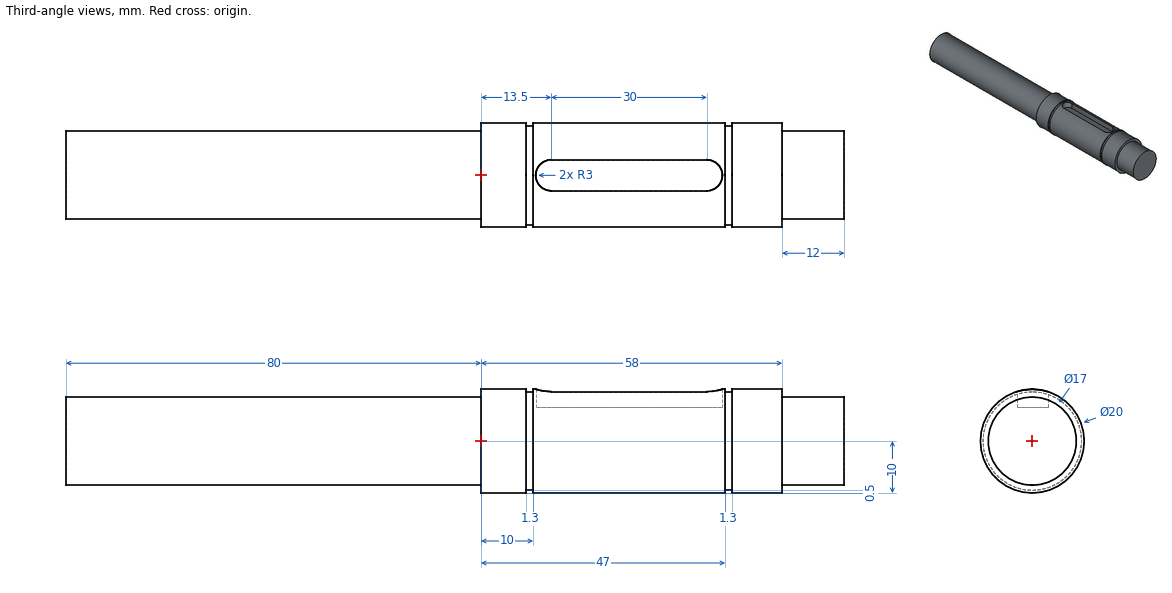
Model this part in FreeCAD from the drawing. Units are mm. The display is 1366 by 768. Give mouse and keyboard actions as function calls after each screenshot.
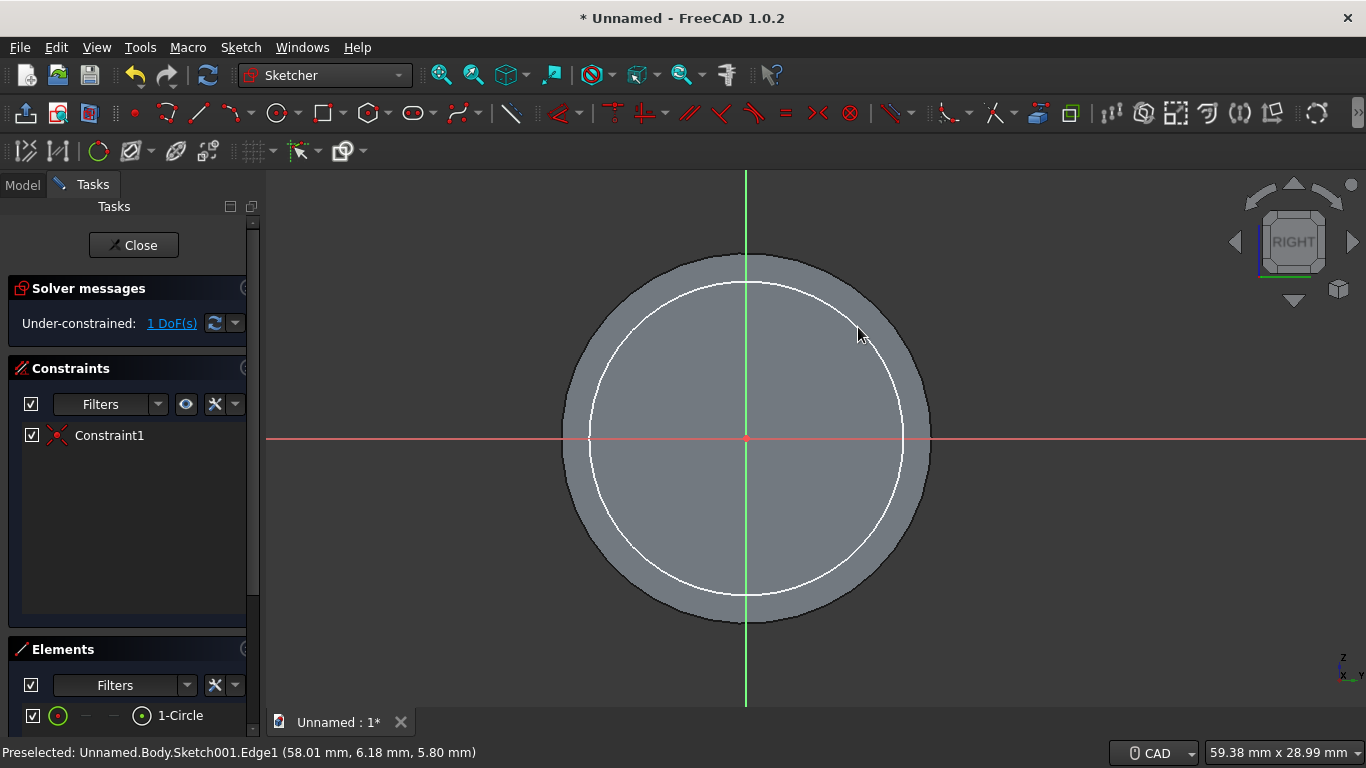
click(558, 114)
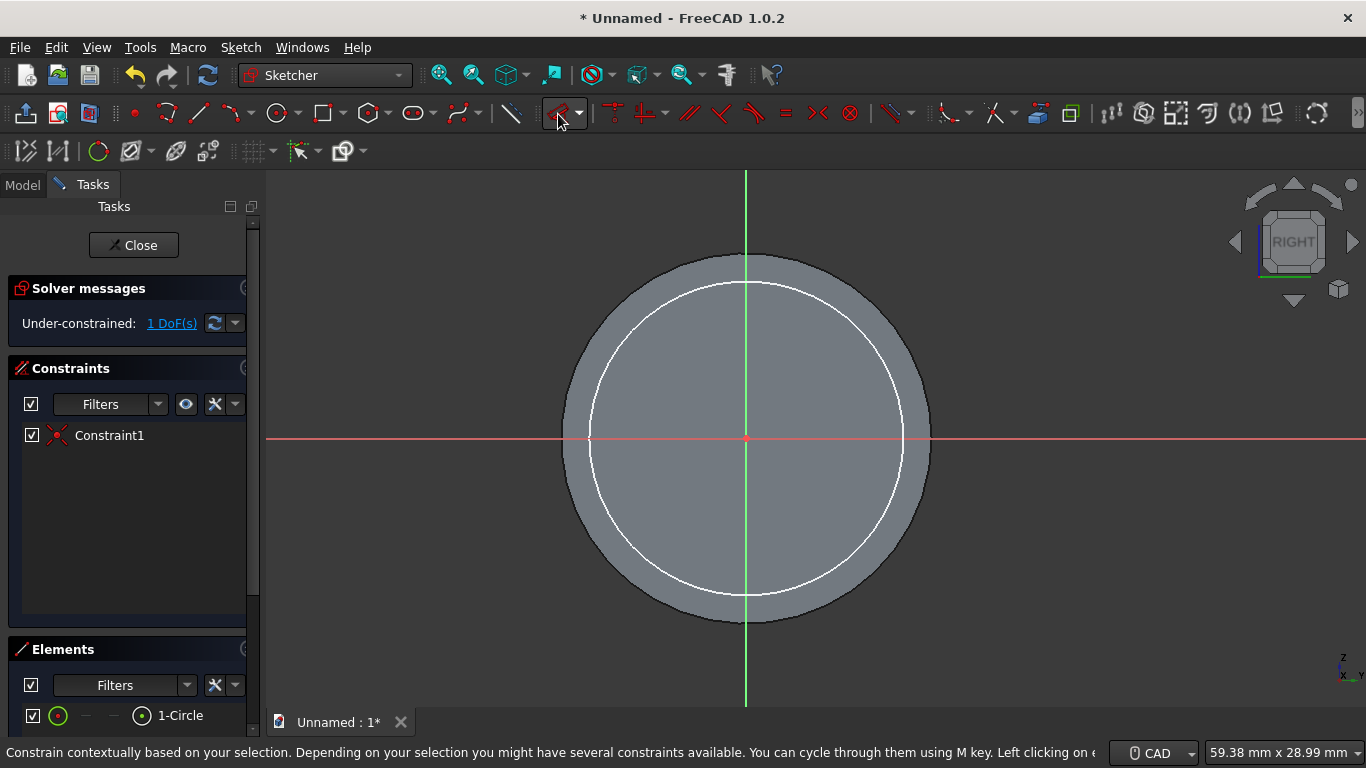
click(857, 327)
click(880, 304)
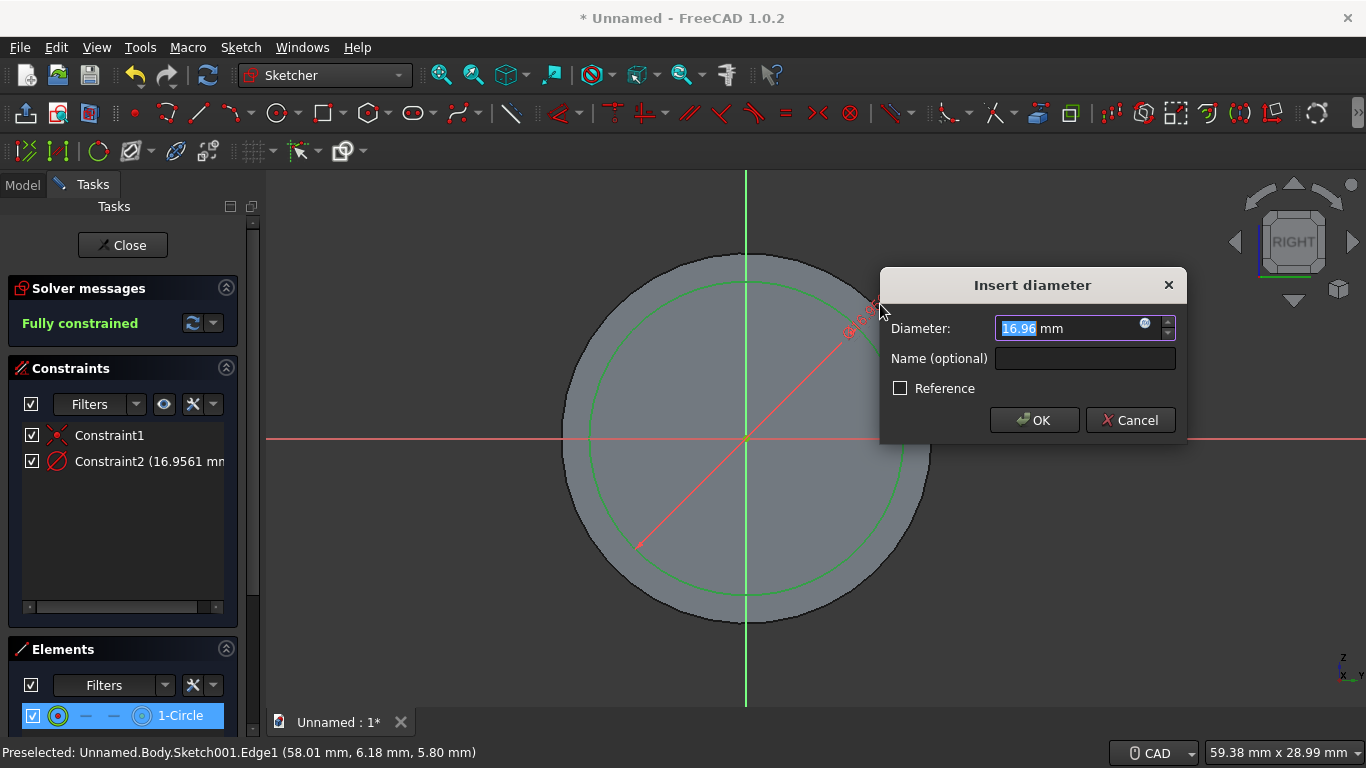
text(17)
key(Return)
key(Escape)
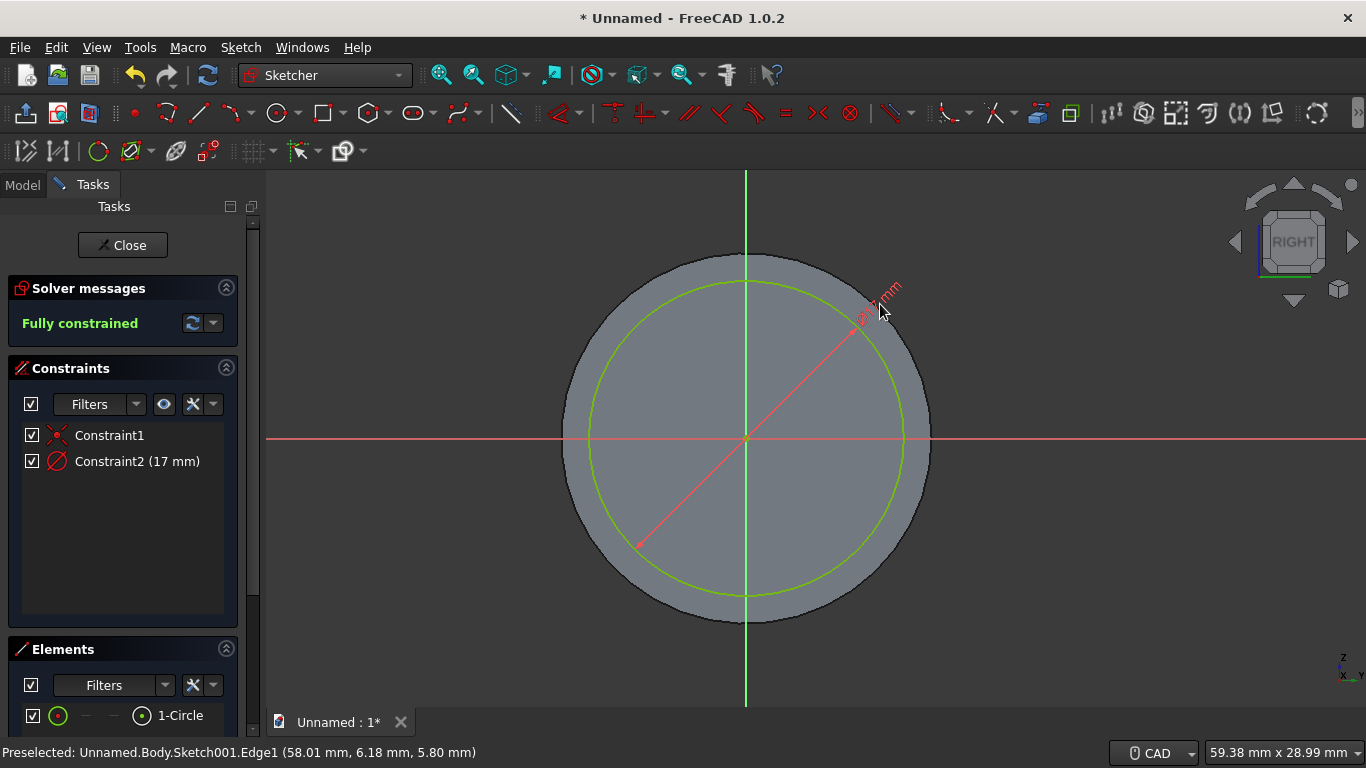
click(123, 245)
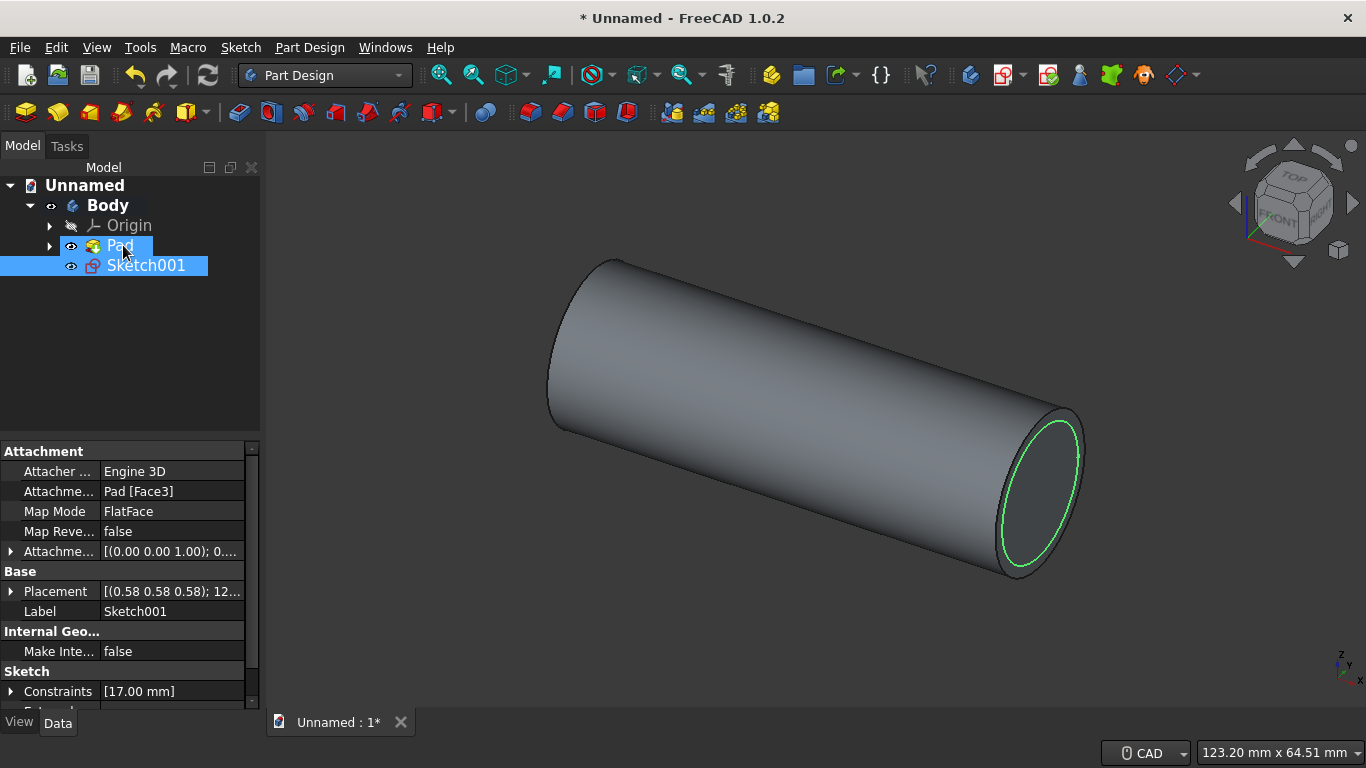
click(26, 112)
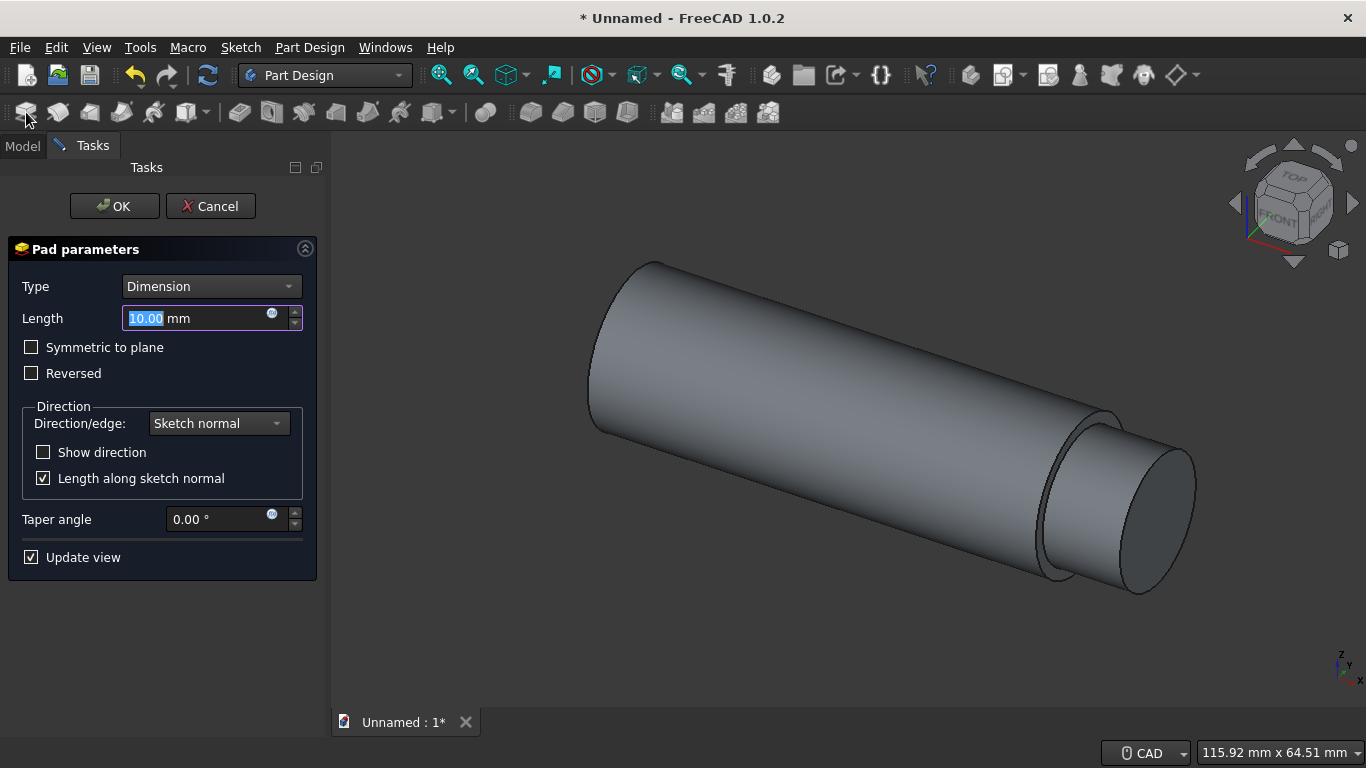
text(12)
key(Tab)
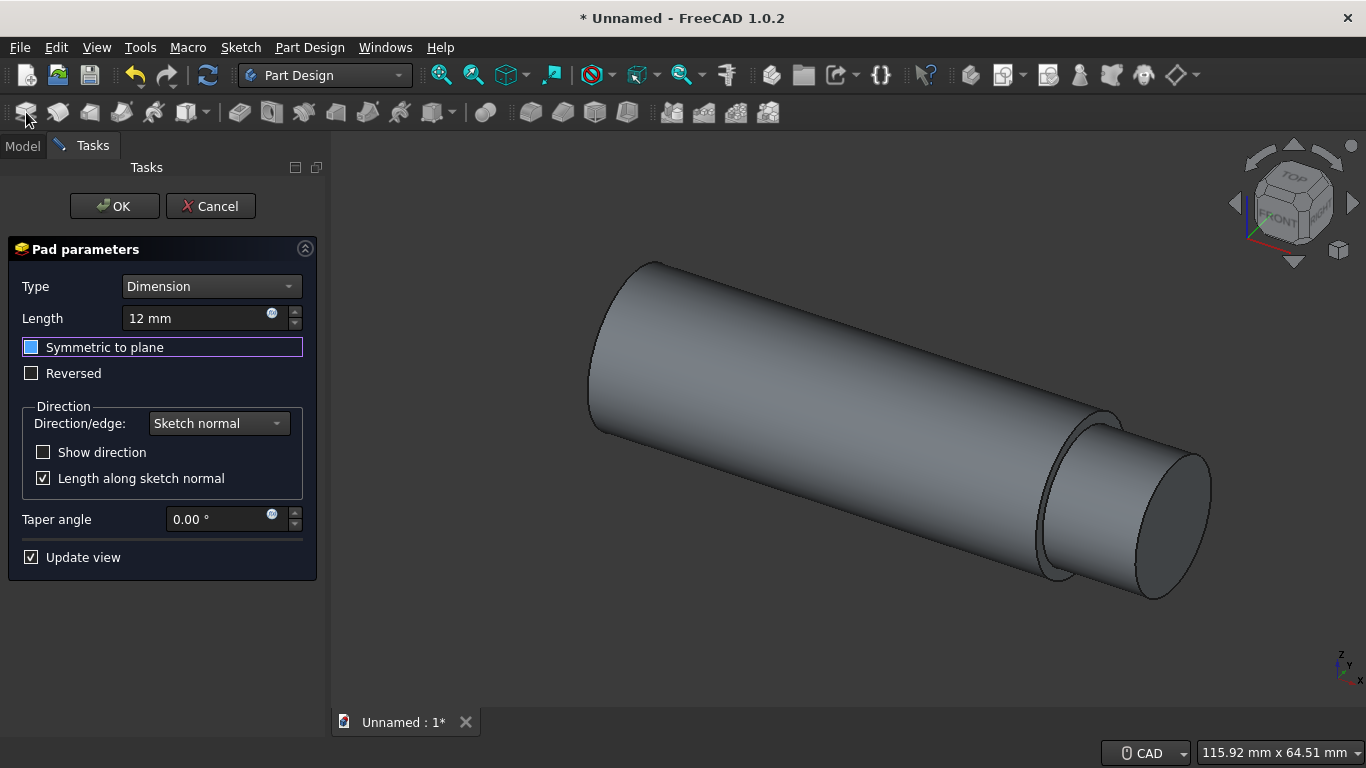
click(115, 206)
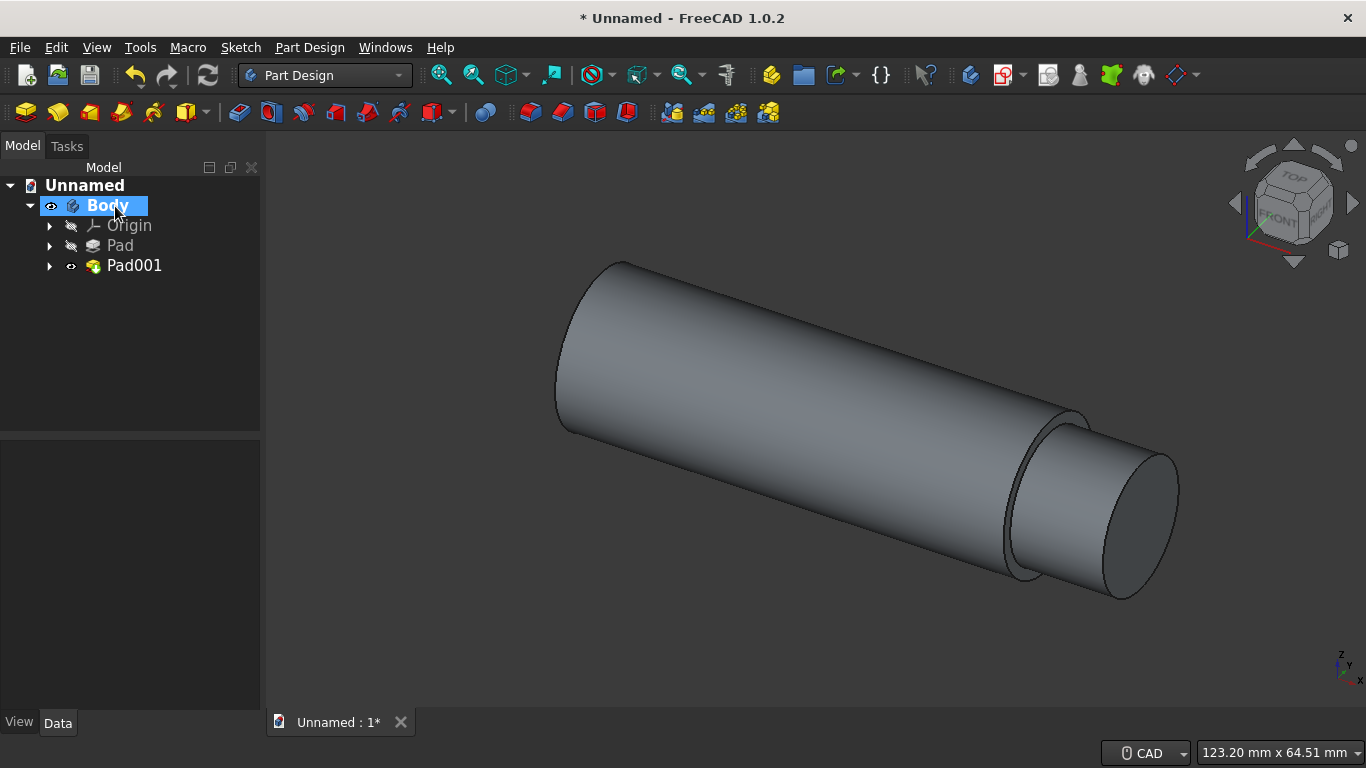
click(50, 226)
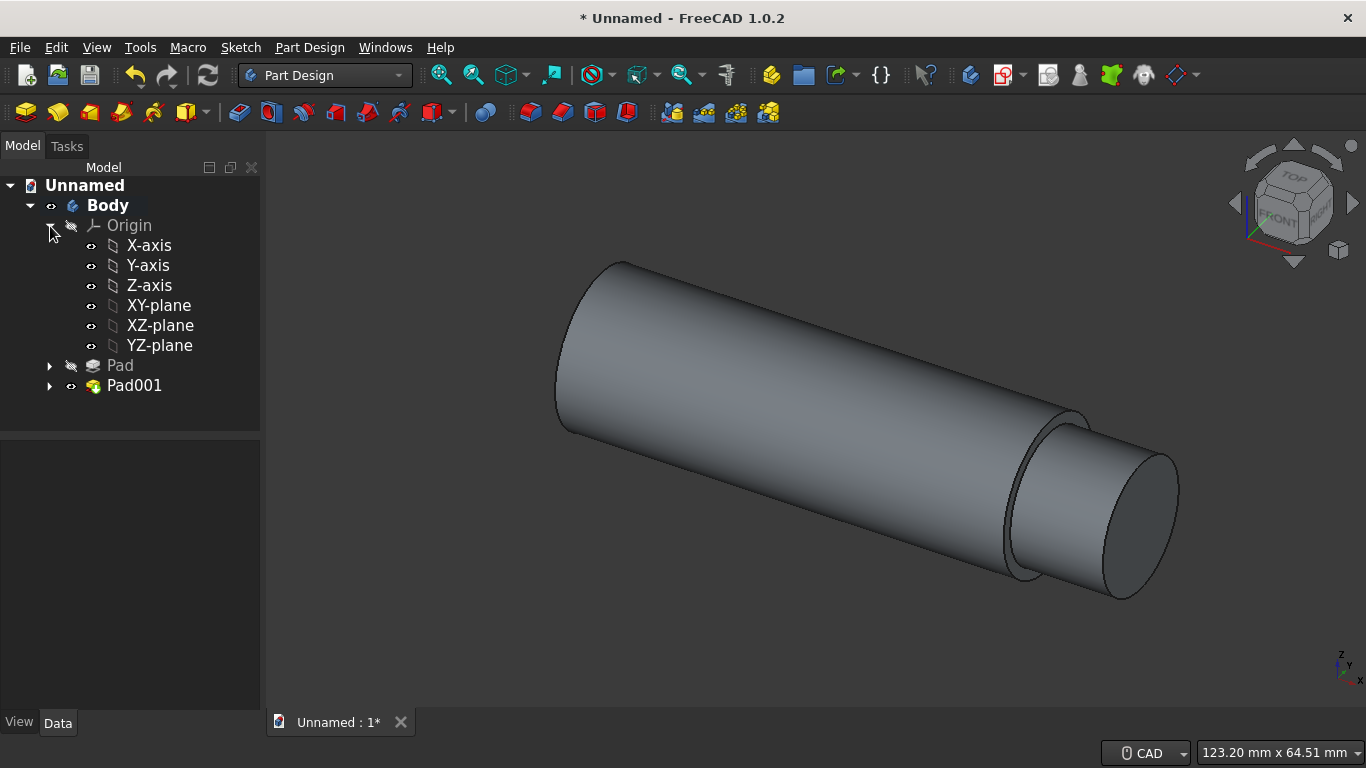
click(136, 346)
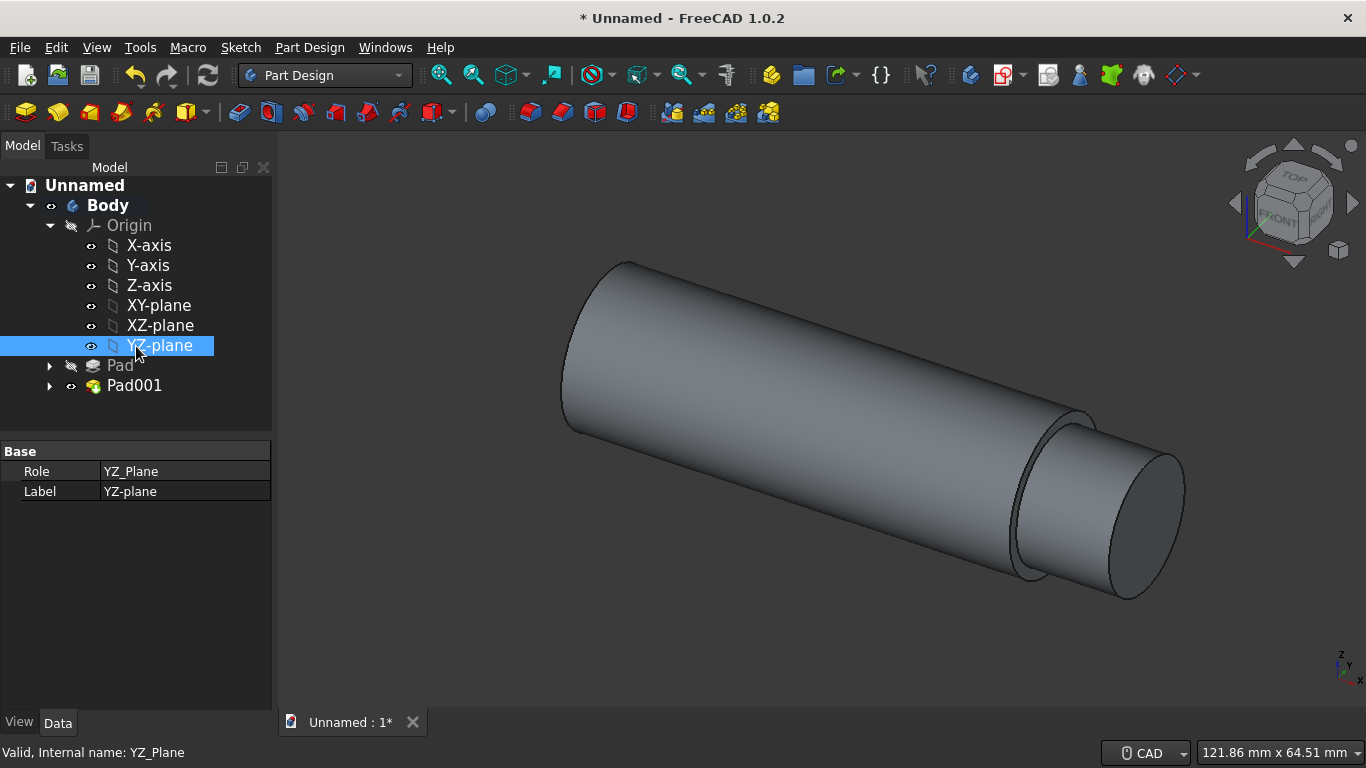
click(1176, 76)